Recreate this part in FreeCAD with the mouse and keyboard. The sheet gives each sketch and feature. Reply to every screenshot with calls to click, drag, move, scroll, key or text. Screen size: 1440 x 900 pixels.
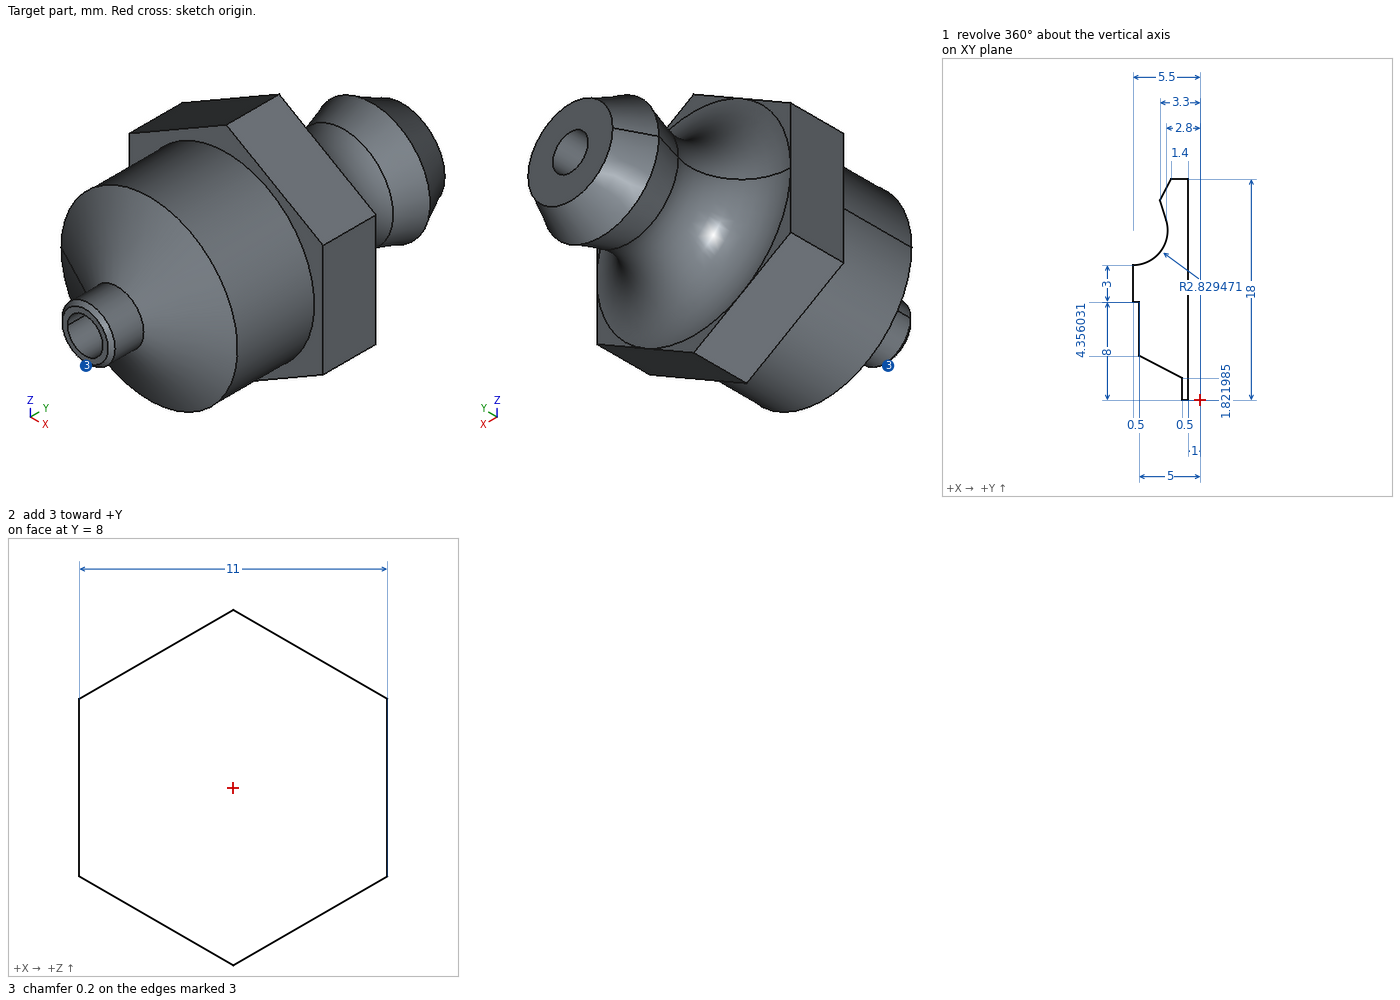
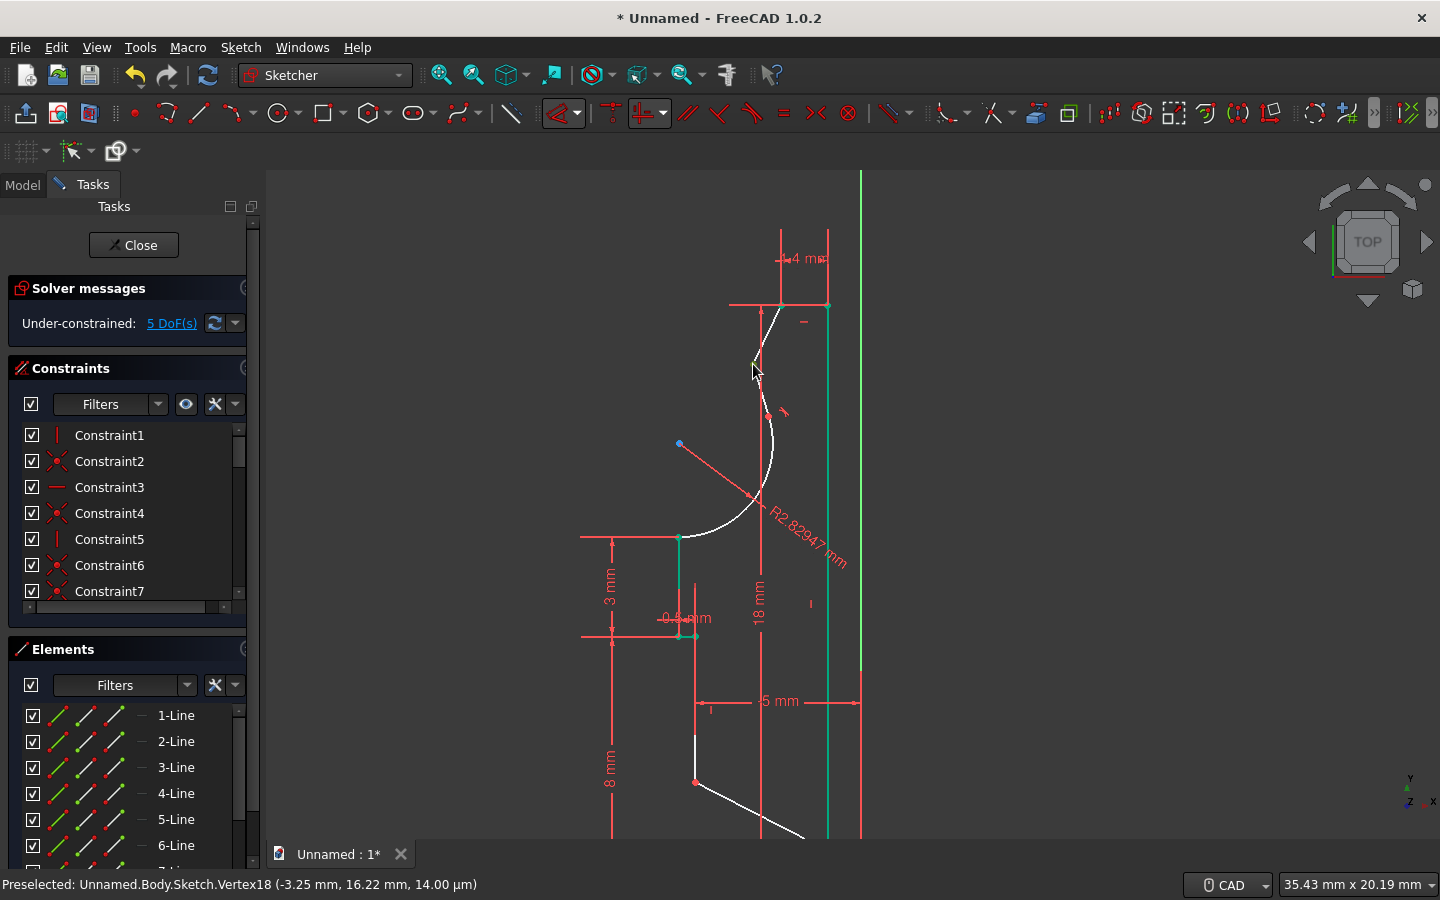
key(l)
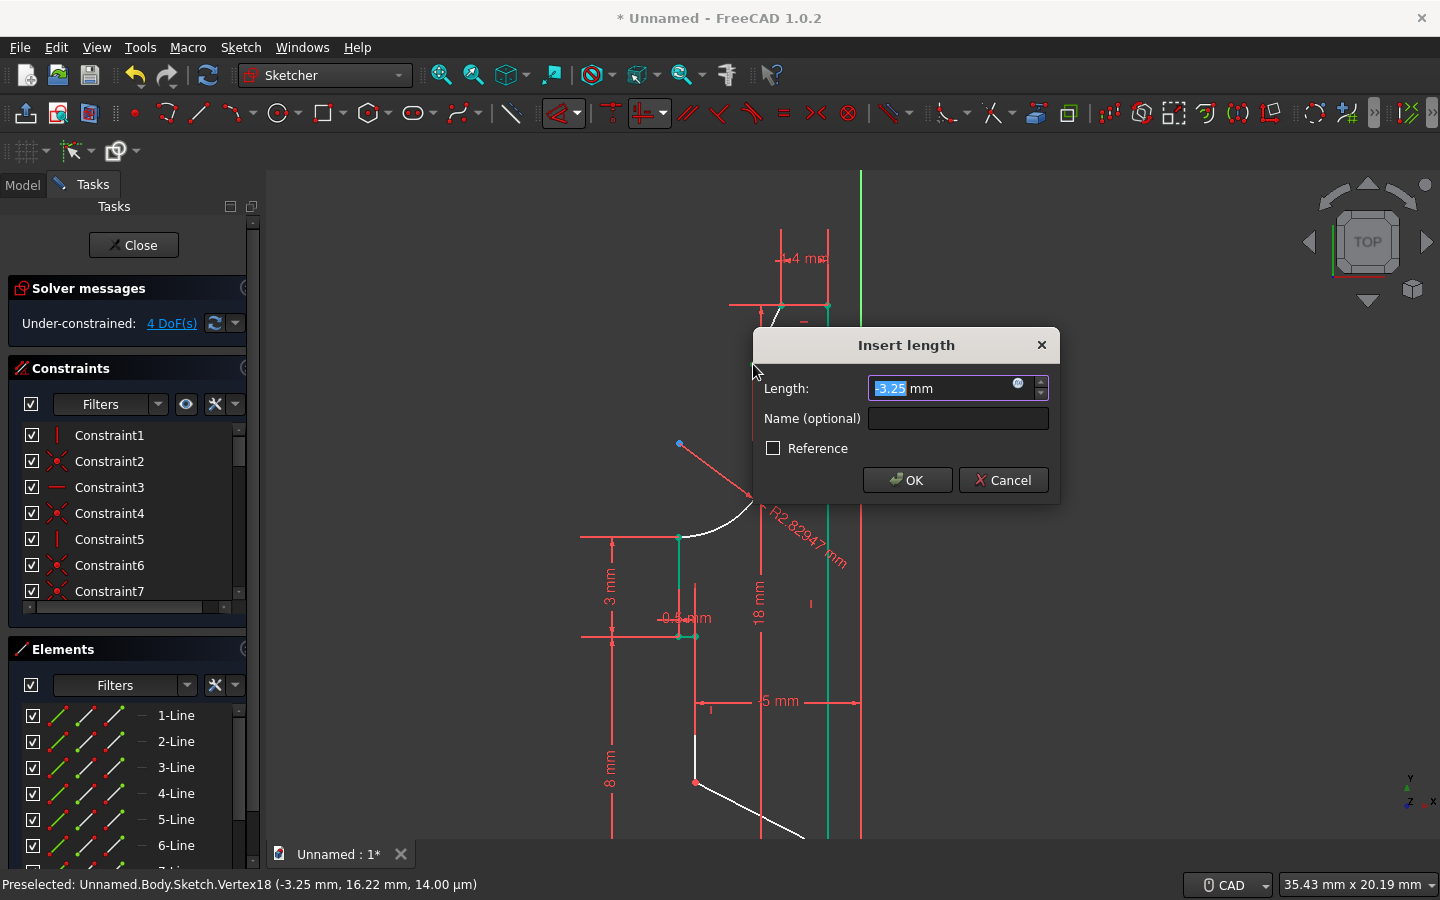
text(-3.3)
key(Return)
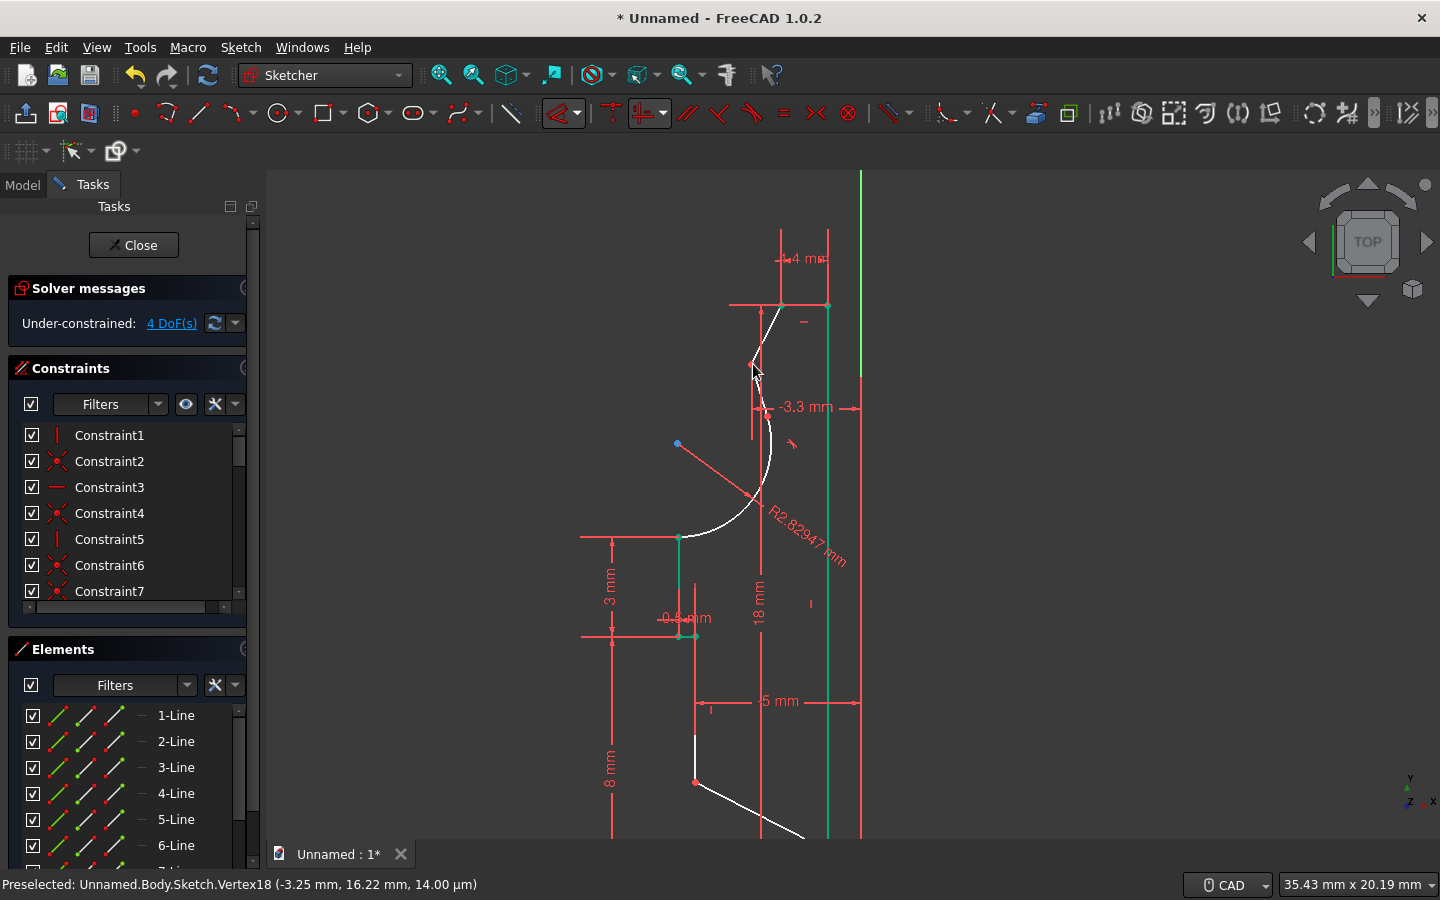
click(767, 416)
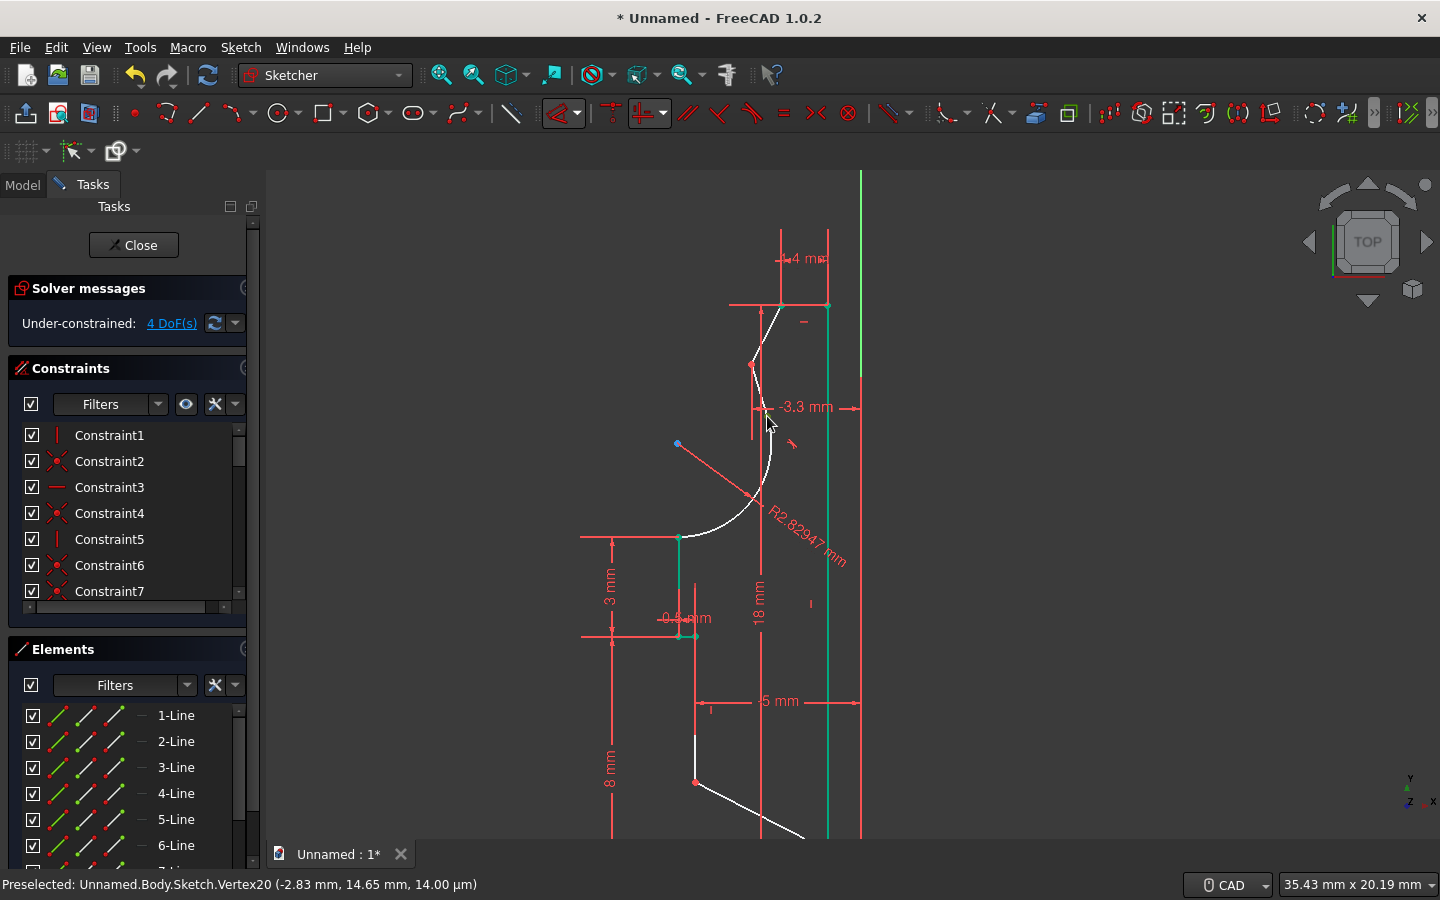
key(l)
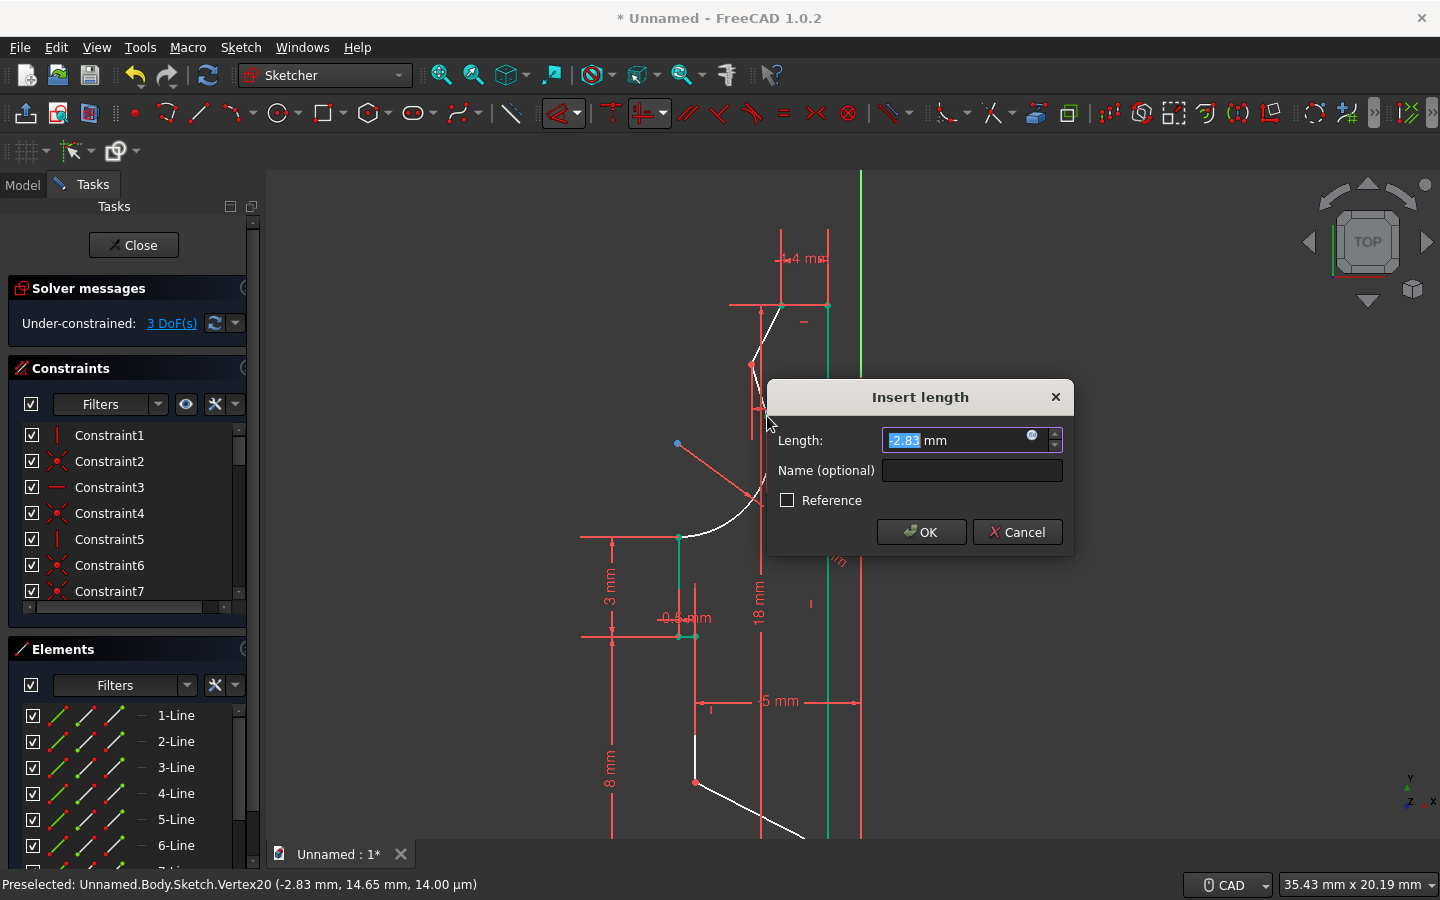
text(-2.8)
key(Return)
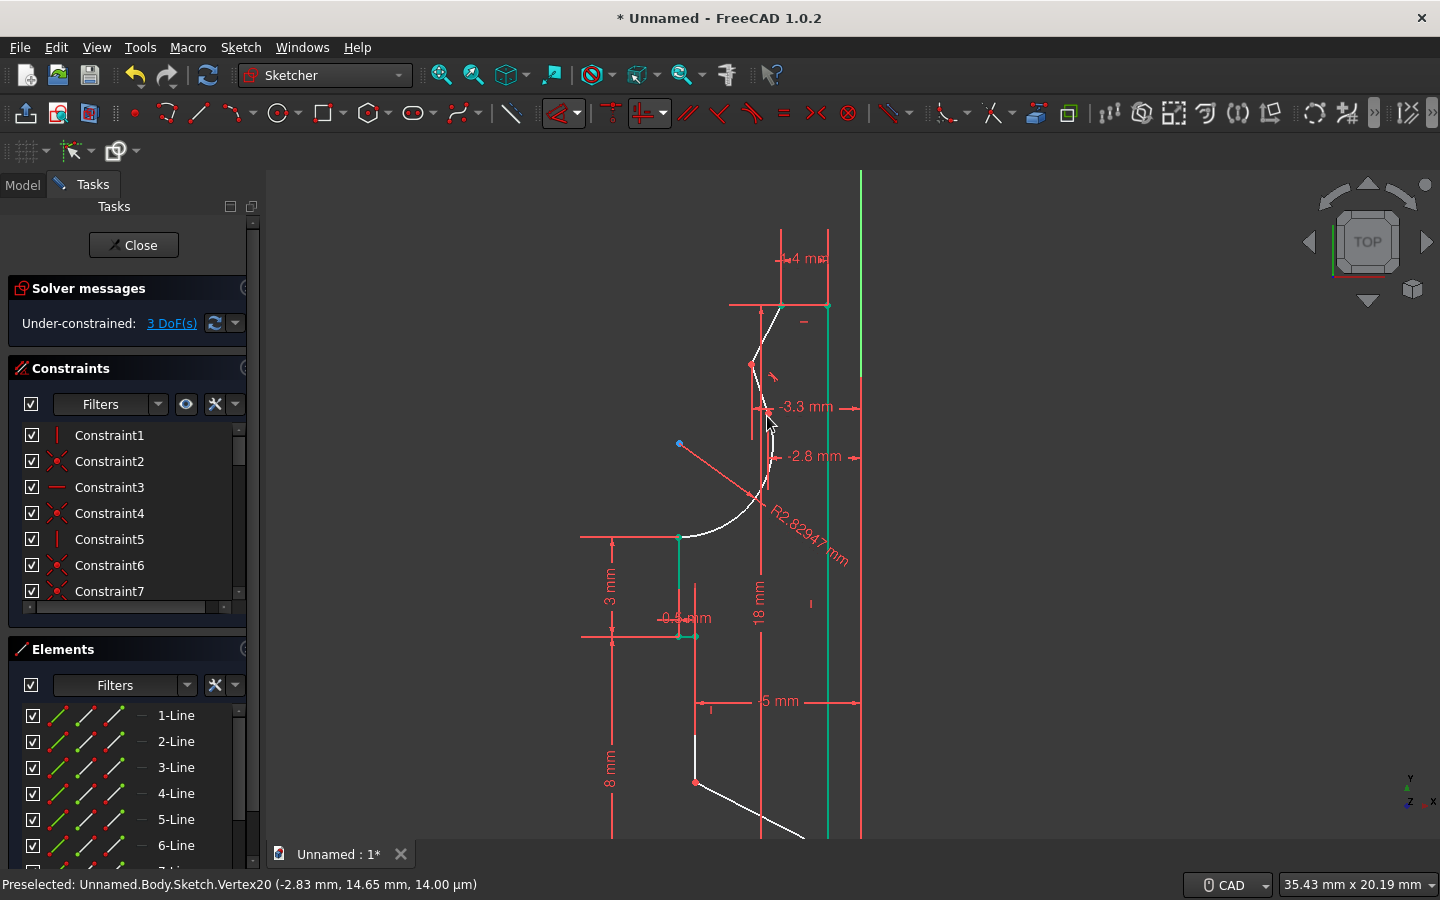
click(679, 443)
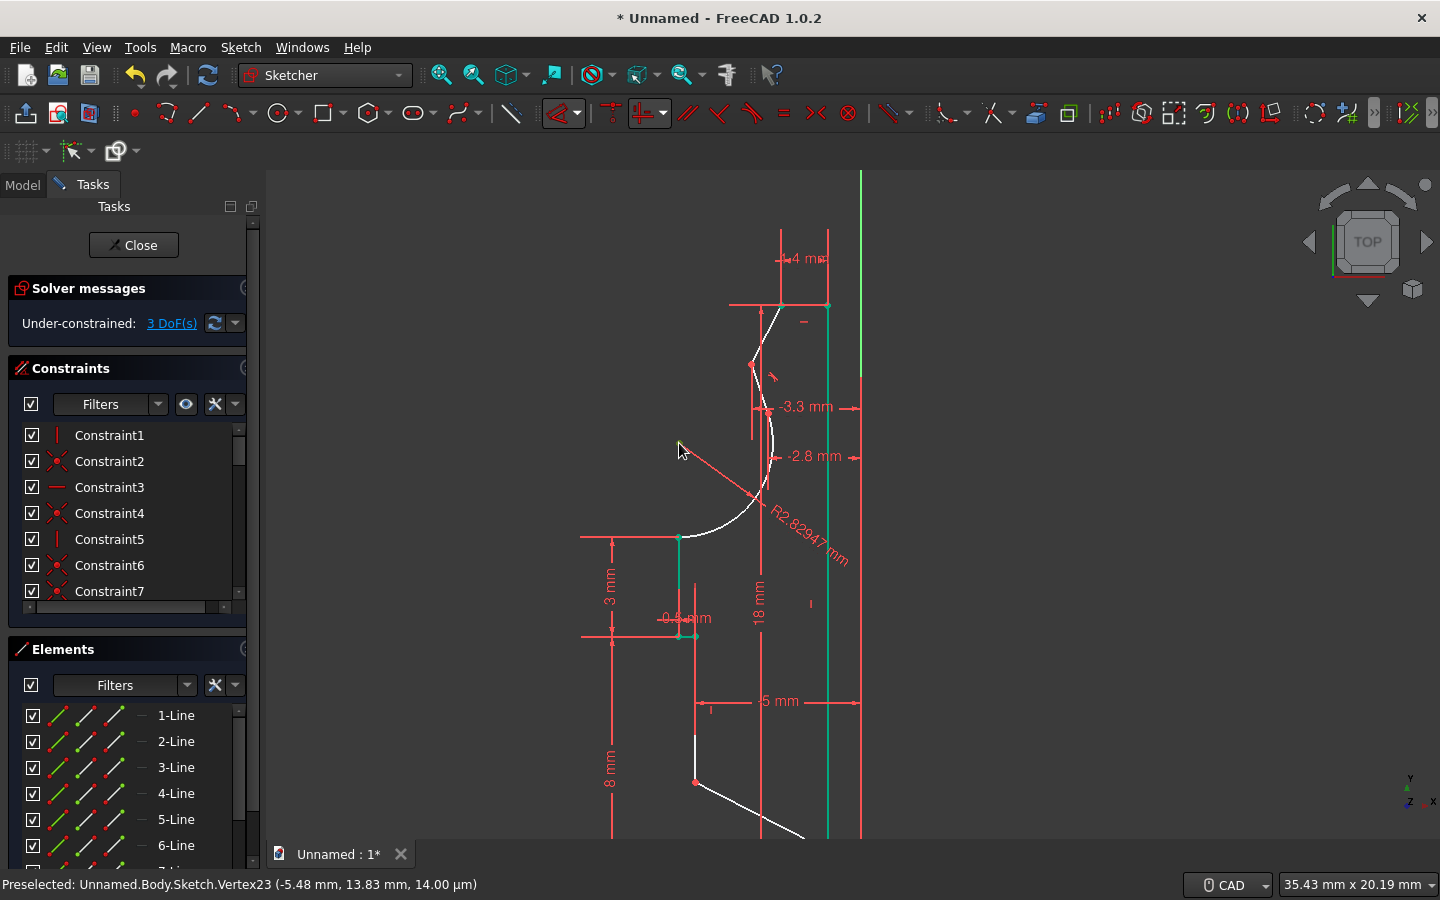
click(580, 114)